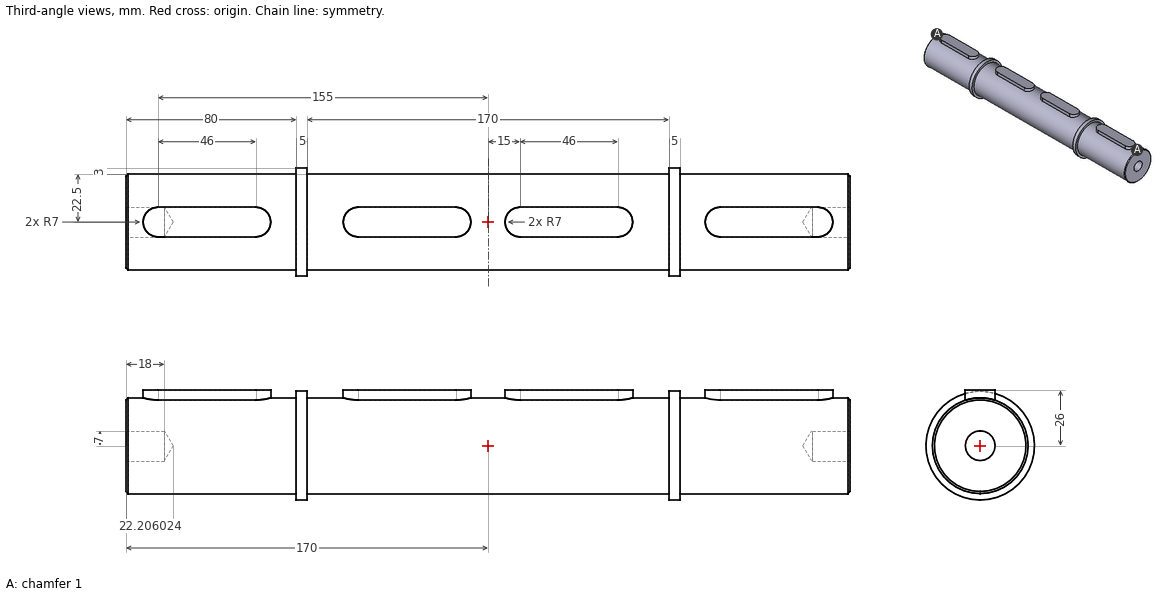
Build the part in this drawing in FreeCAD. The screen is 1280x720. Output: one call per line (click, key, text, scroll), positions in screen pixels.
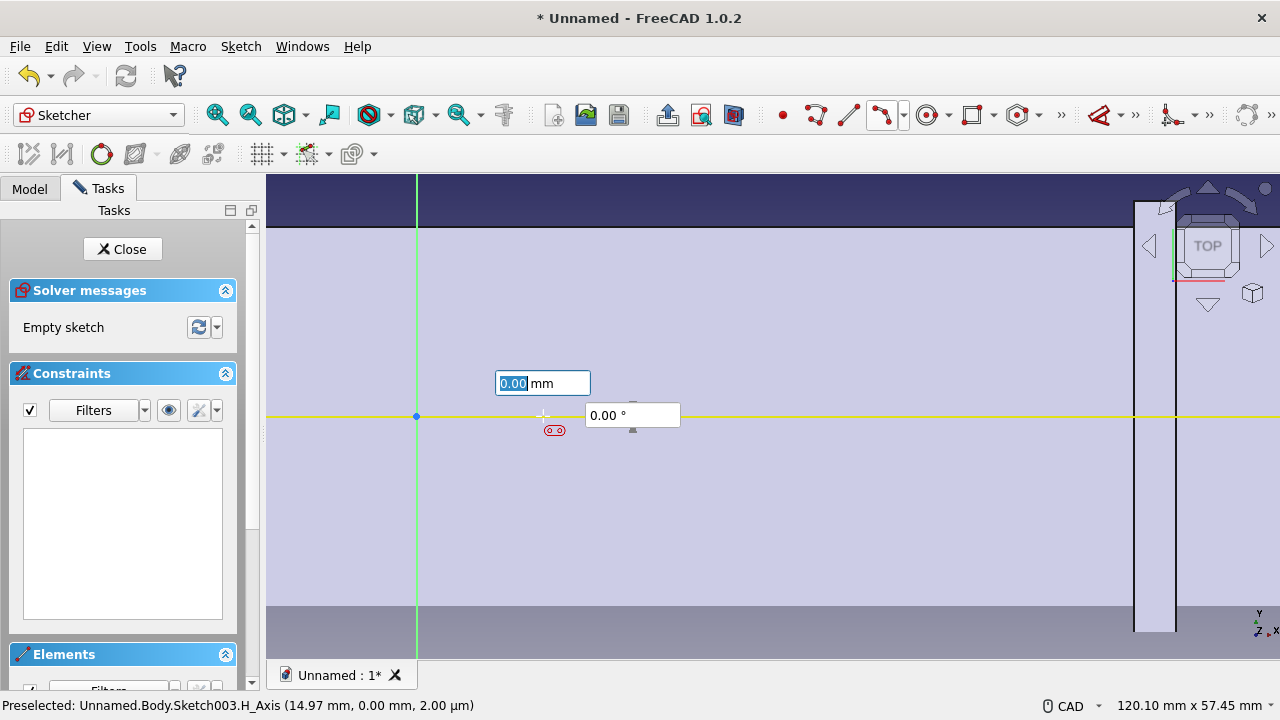
click(932, 407)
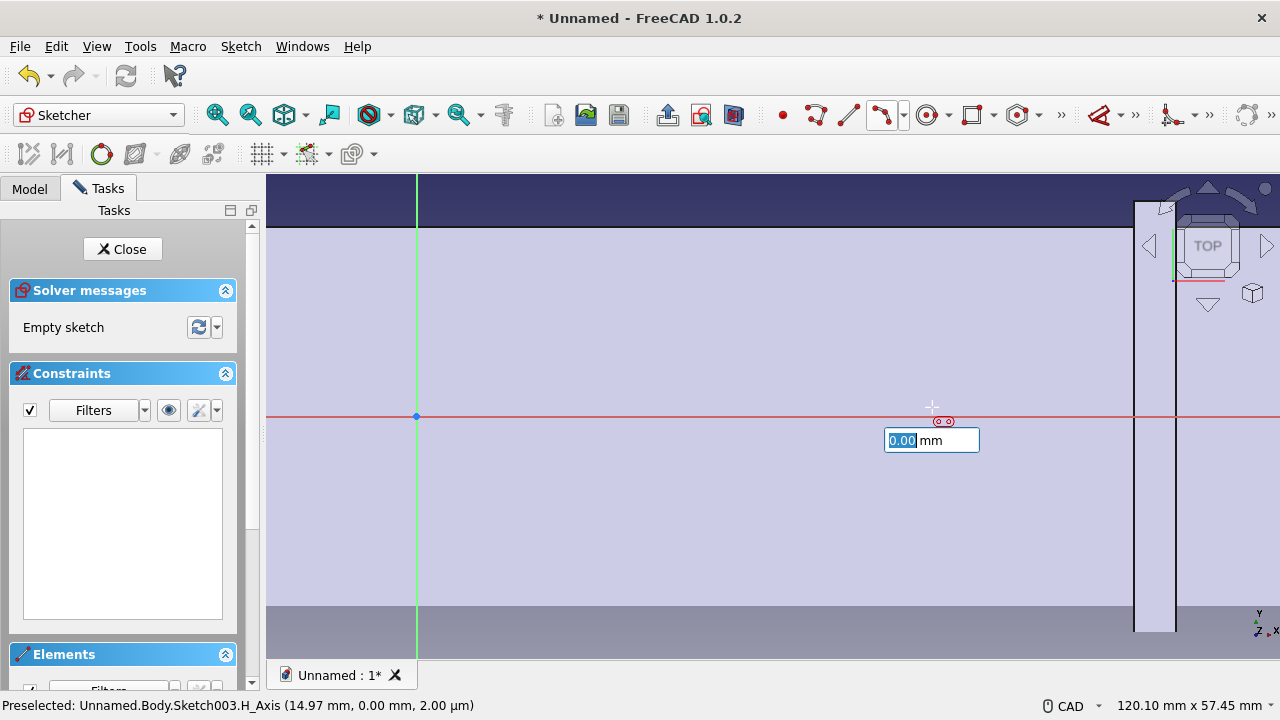
click(737, 357)
key(Escape)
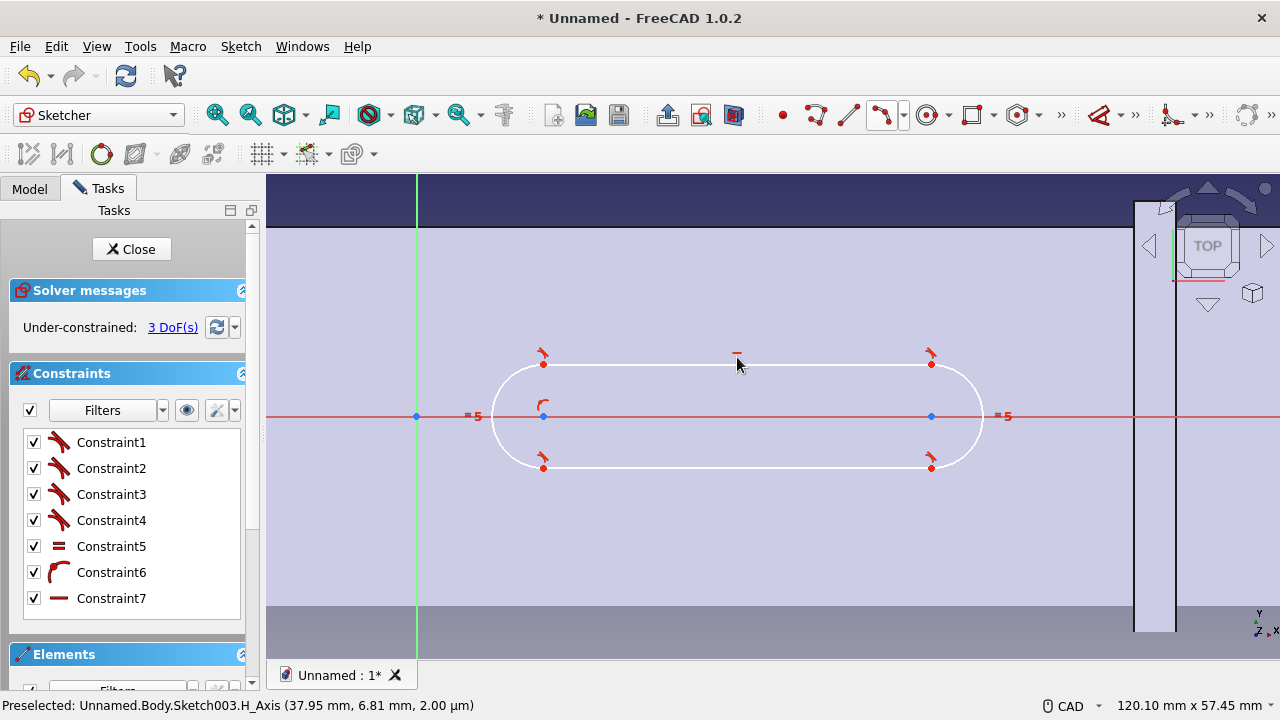
click(1098, 116)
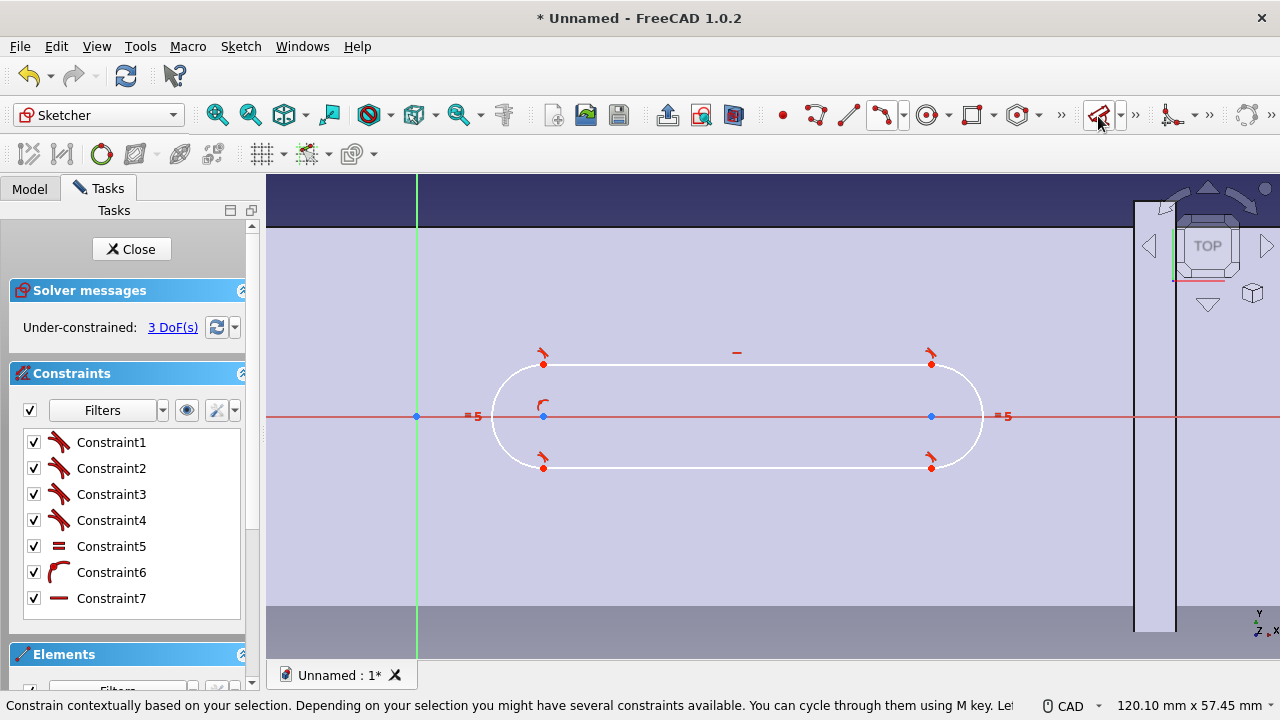
click(502, 386)
click(476, 367)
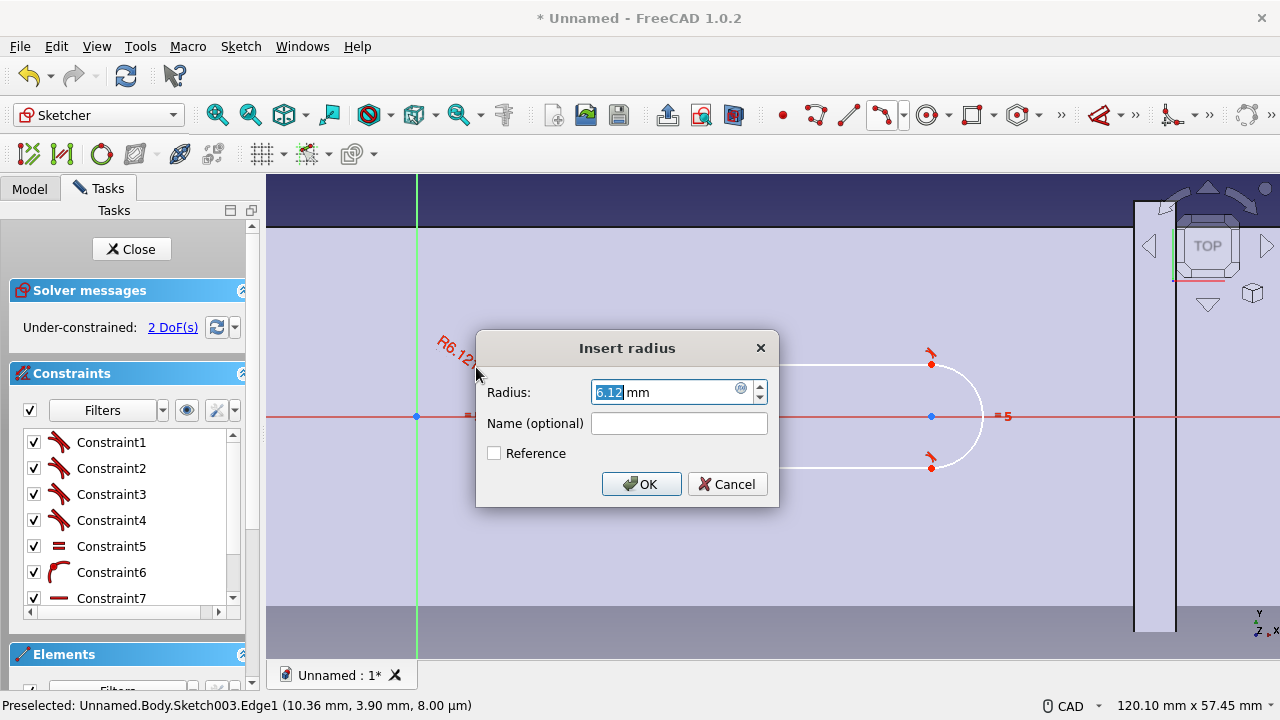
text(7)
key(Return)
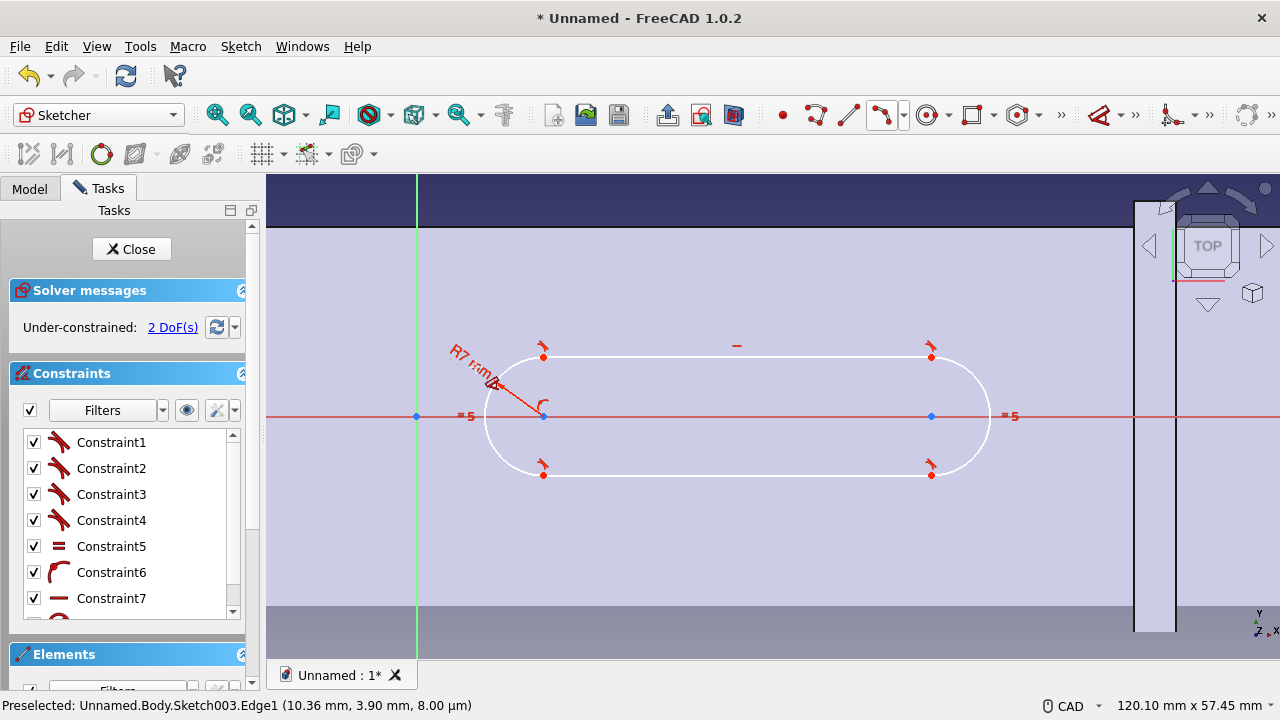
click(660, 357)
click(737, 323)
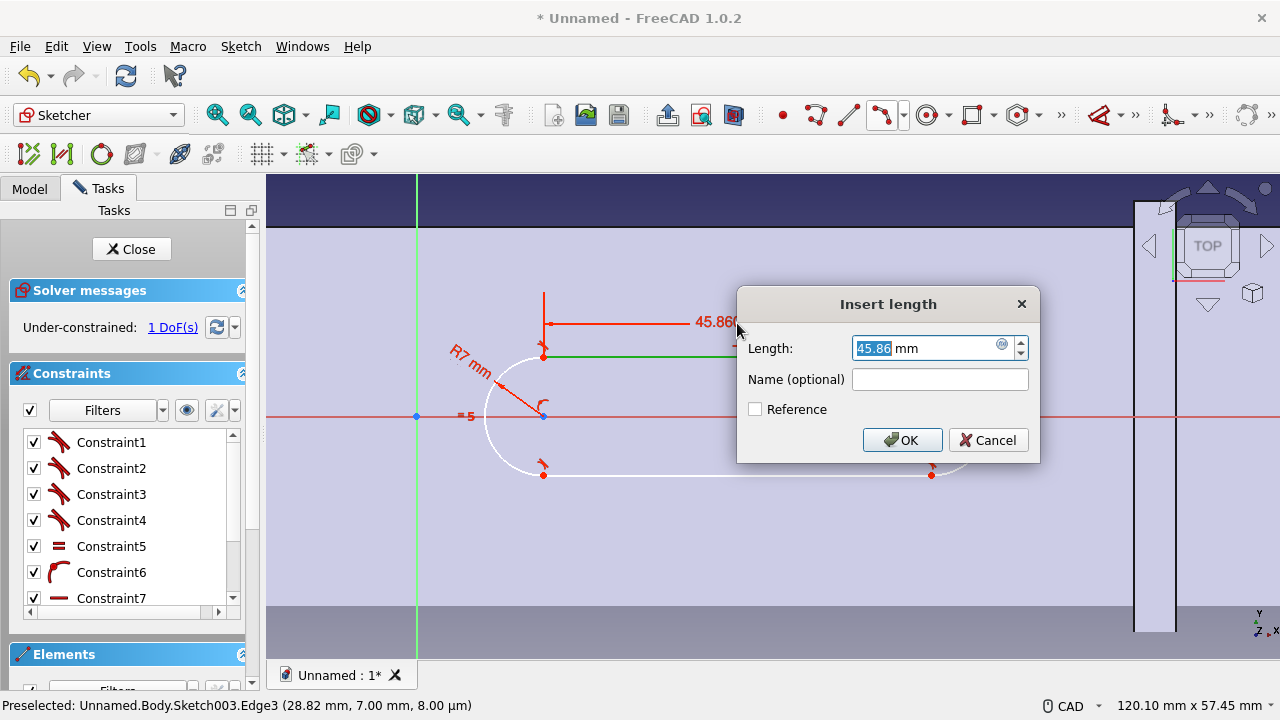
text(46)
key(Return)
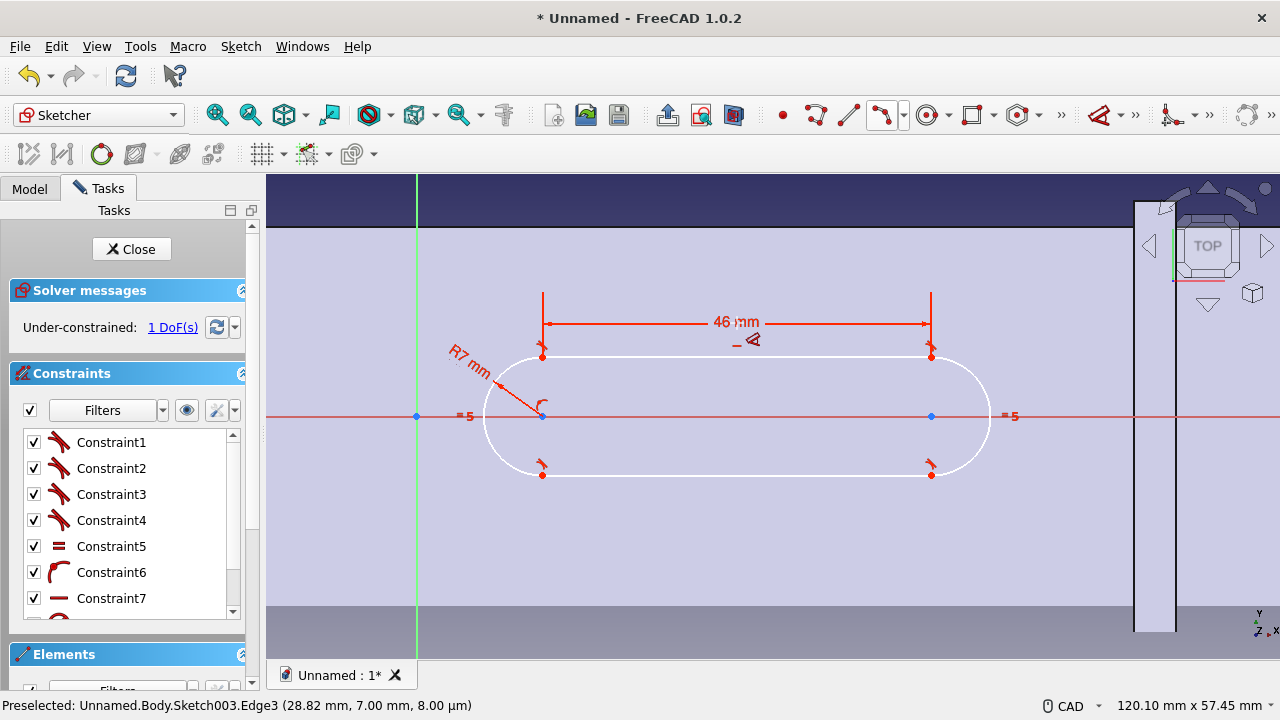
click(543, 357)
click(480, 323)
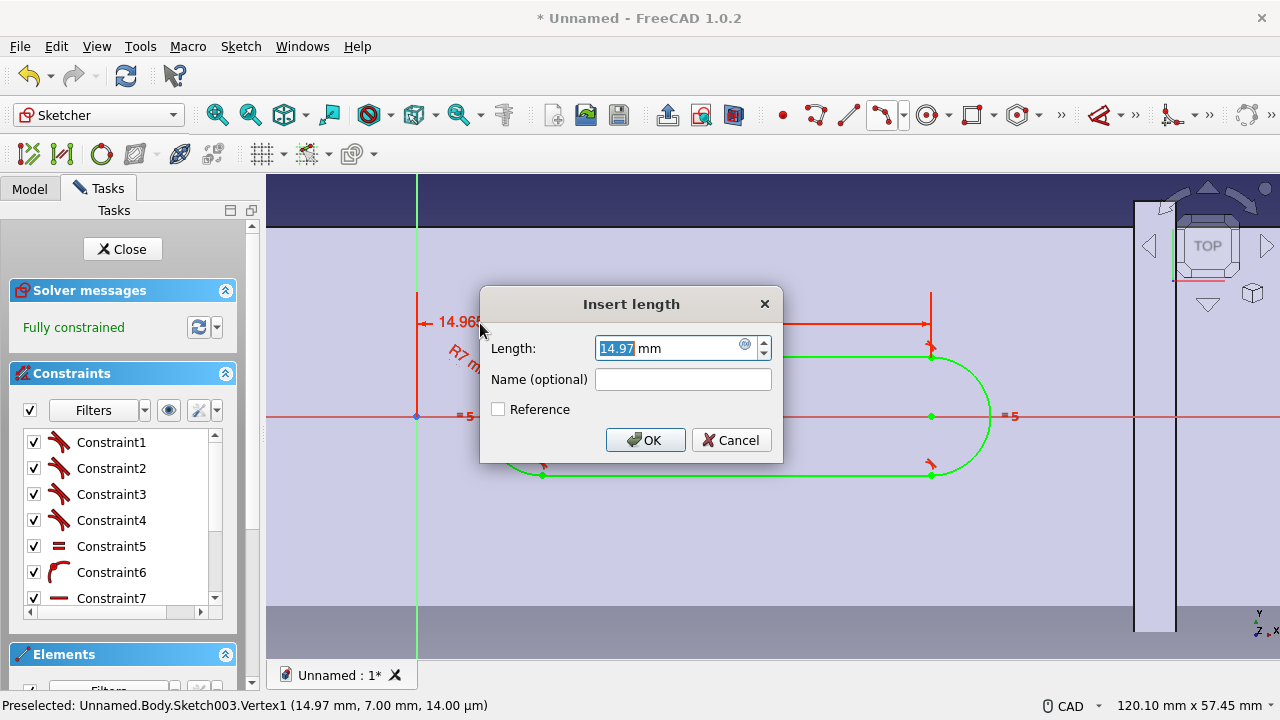
text(15)
key(Return)
key(Escape)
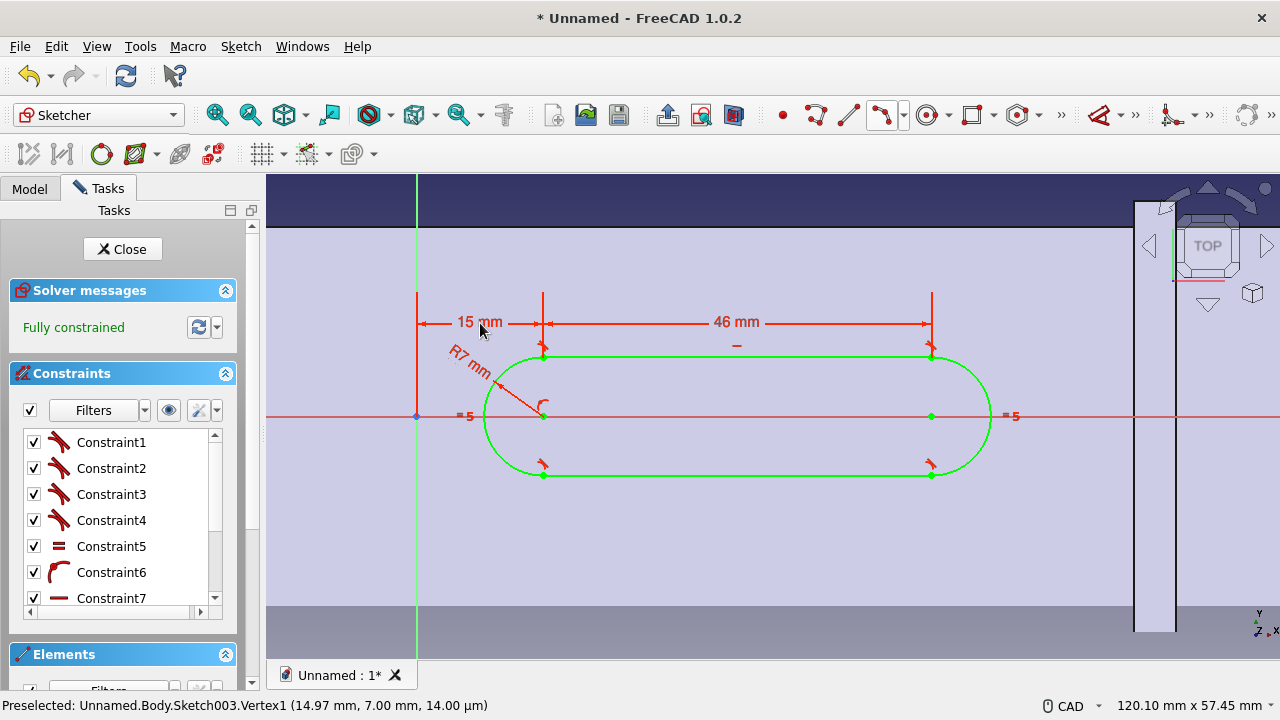
click(123, 249)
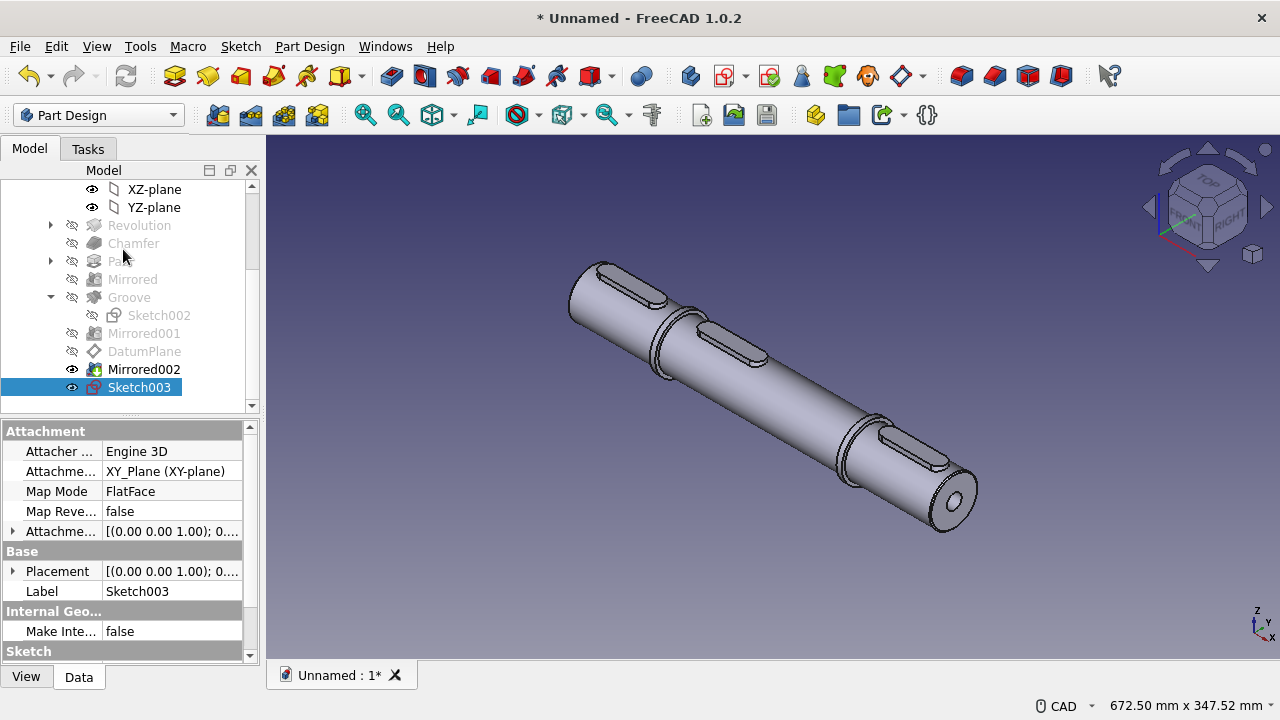
click(175, 76)